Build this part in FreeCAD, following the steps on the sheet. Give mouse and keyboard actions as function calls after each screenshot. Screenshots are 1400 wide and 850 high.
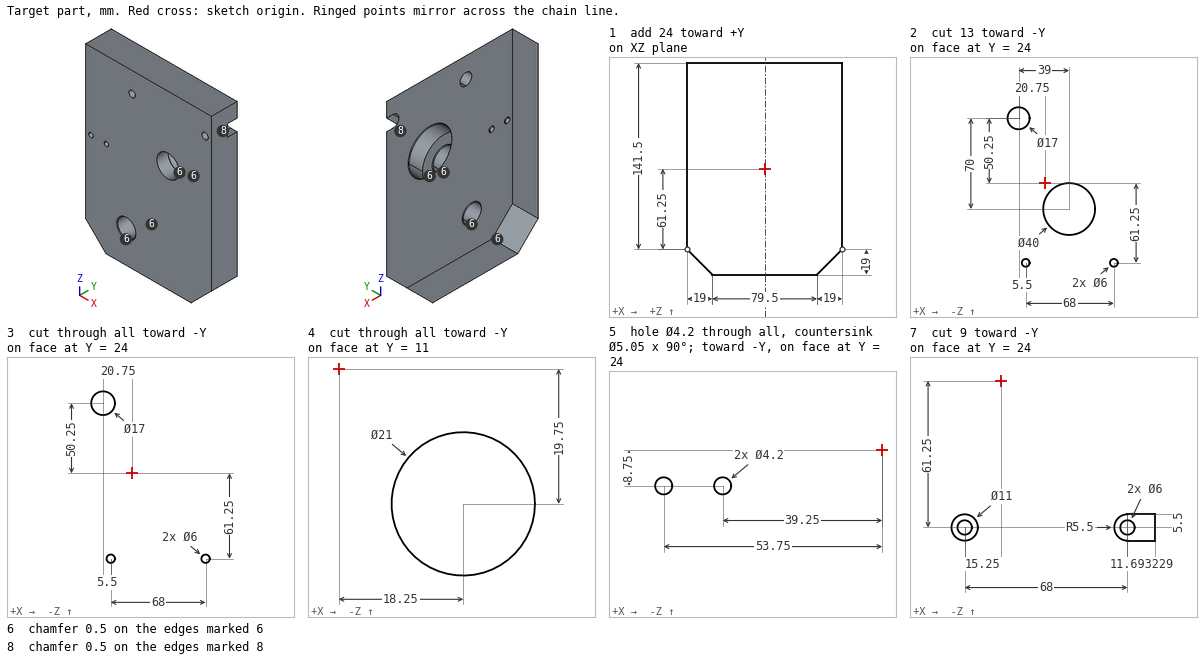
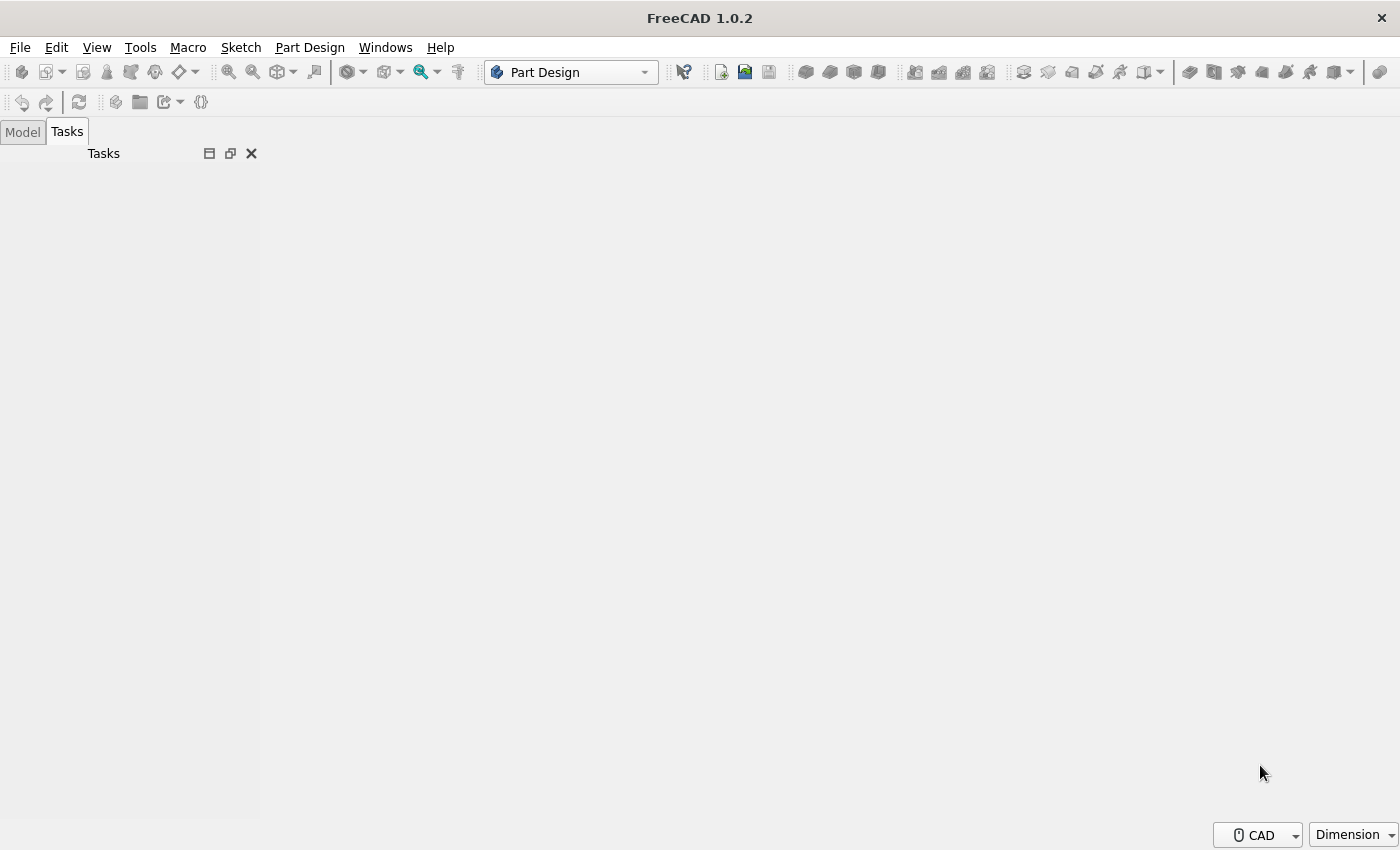
key(ctrl+n)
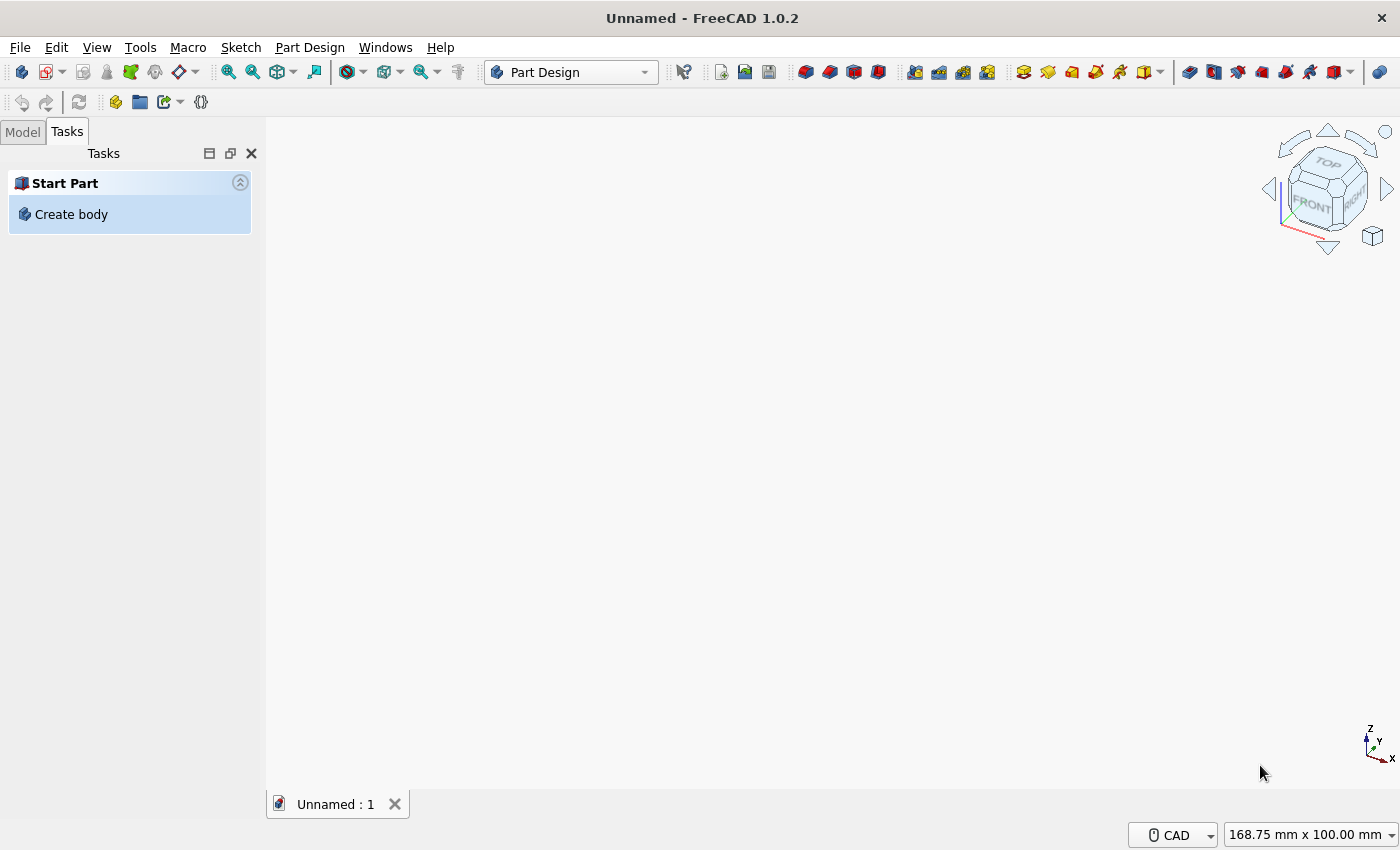
click(46, 72)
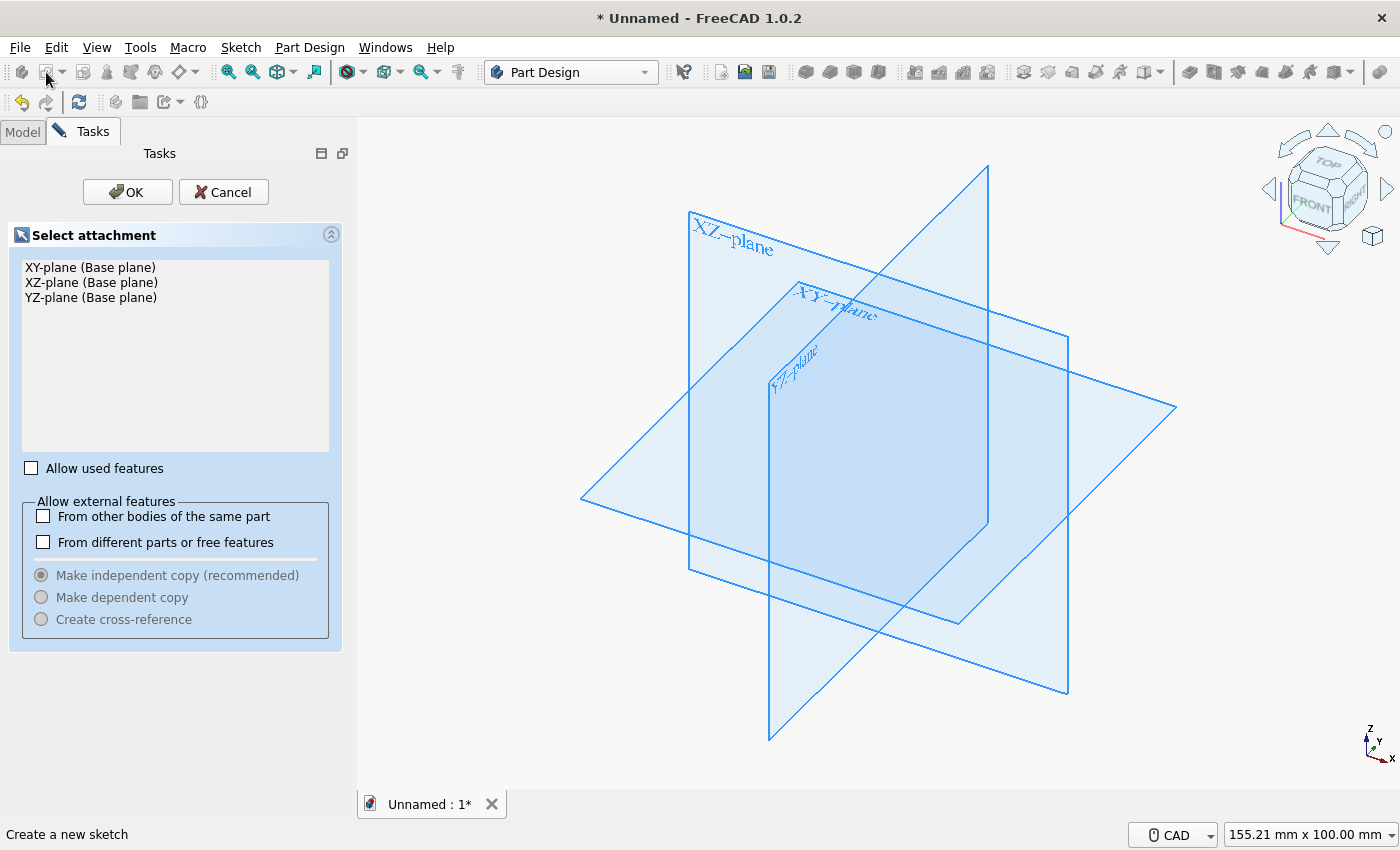
click(82, 282)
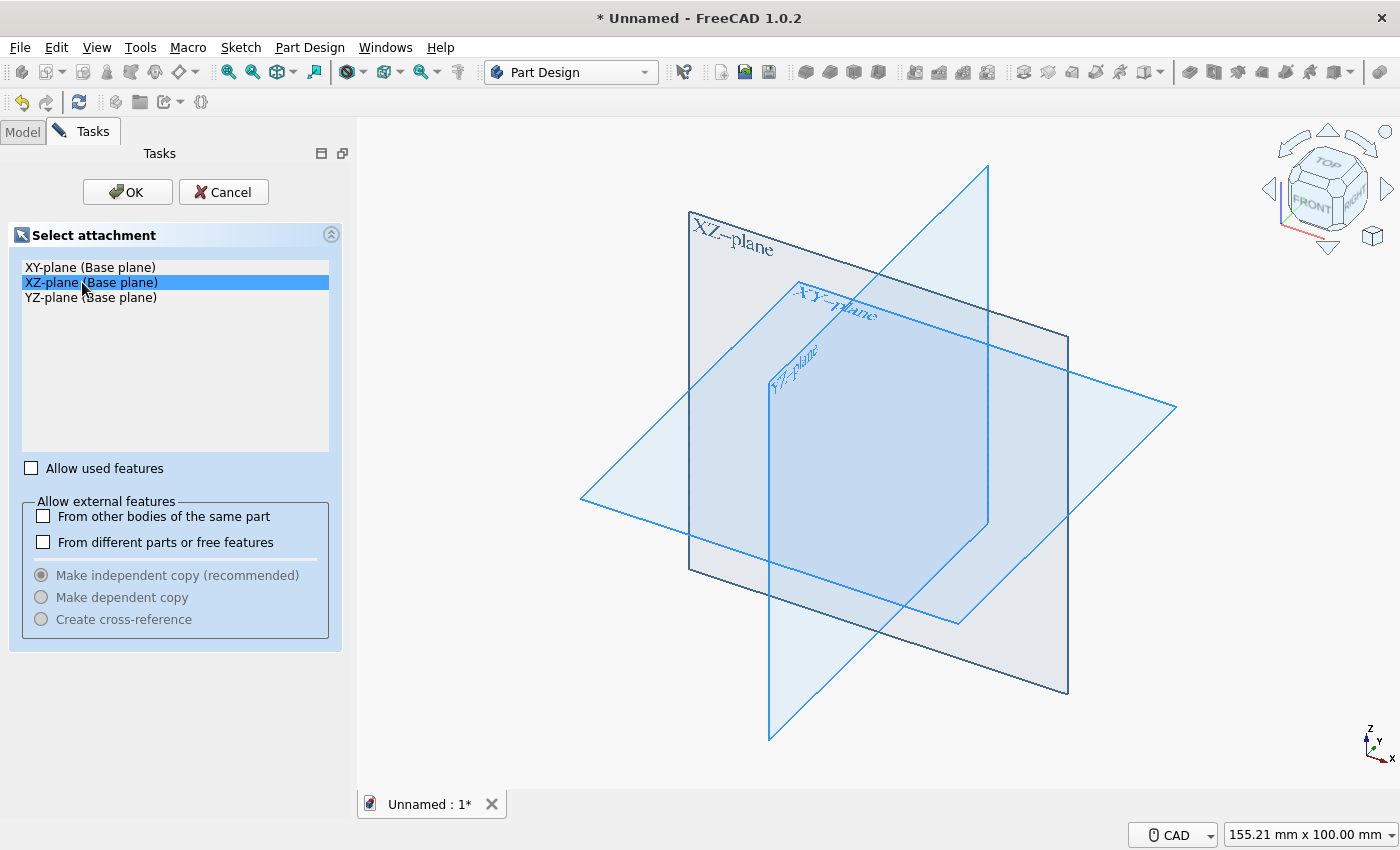
click(128, 192)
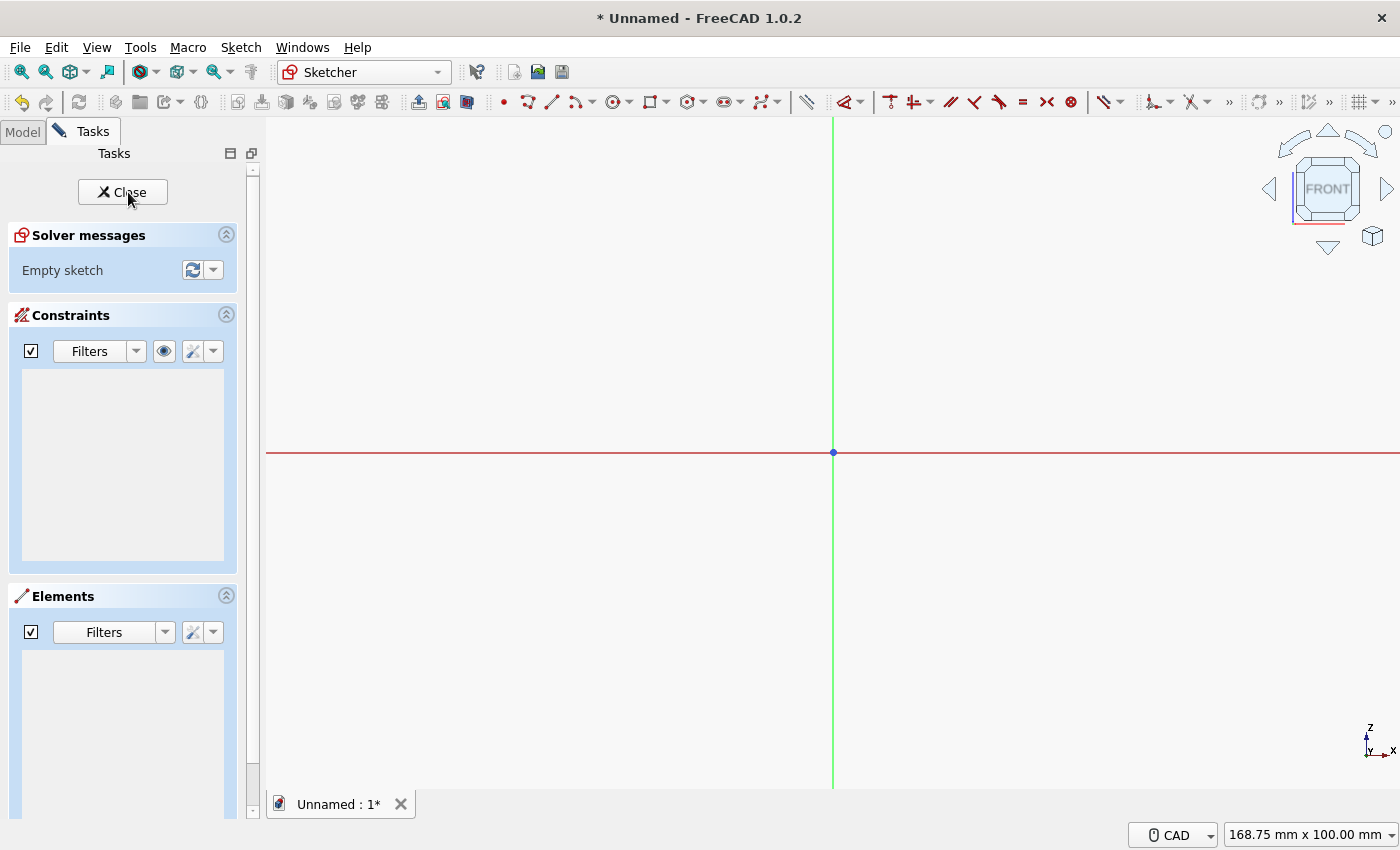
scroll(725, 453, down, 5)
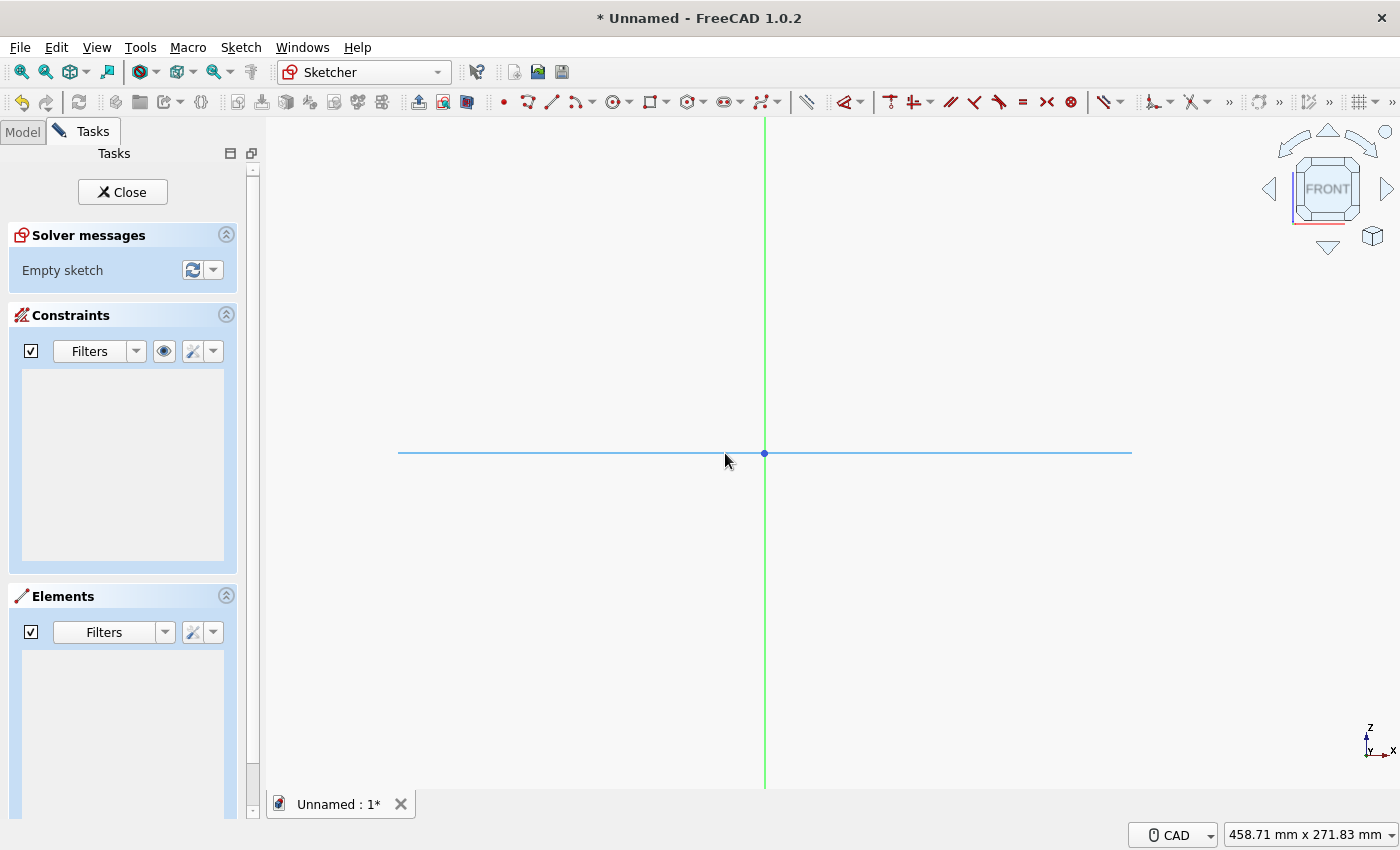
key(g)
key(m)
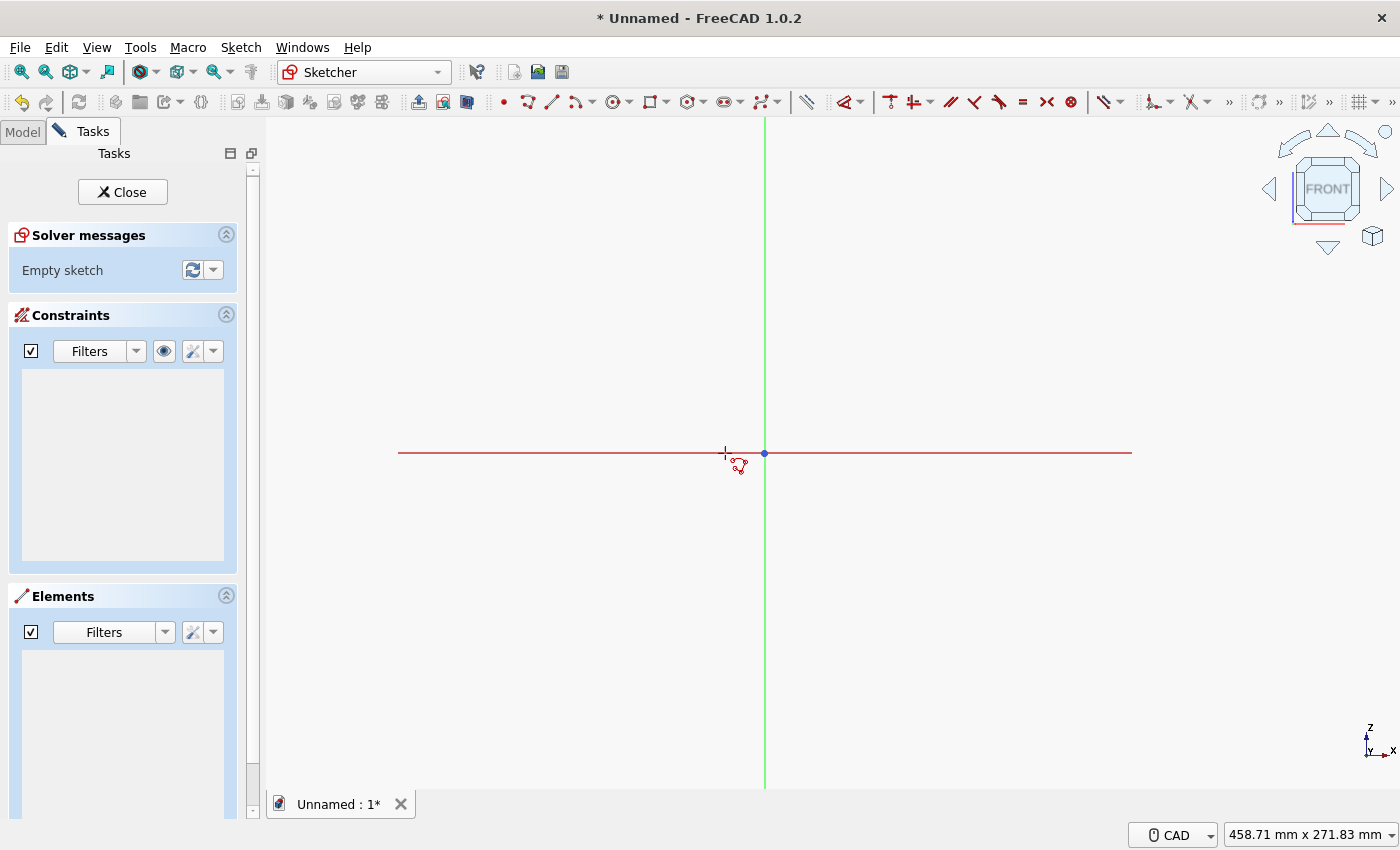
click(620, 605)
click(620, 255)
click(910, 255)
click(910, 605)
click(863, 652)
click(667, 652)
click(620, 606)
key(Escape)
key(Escape)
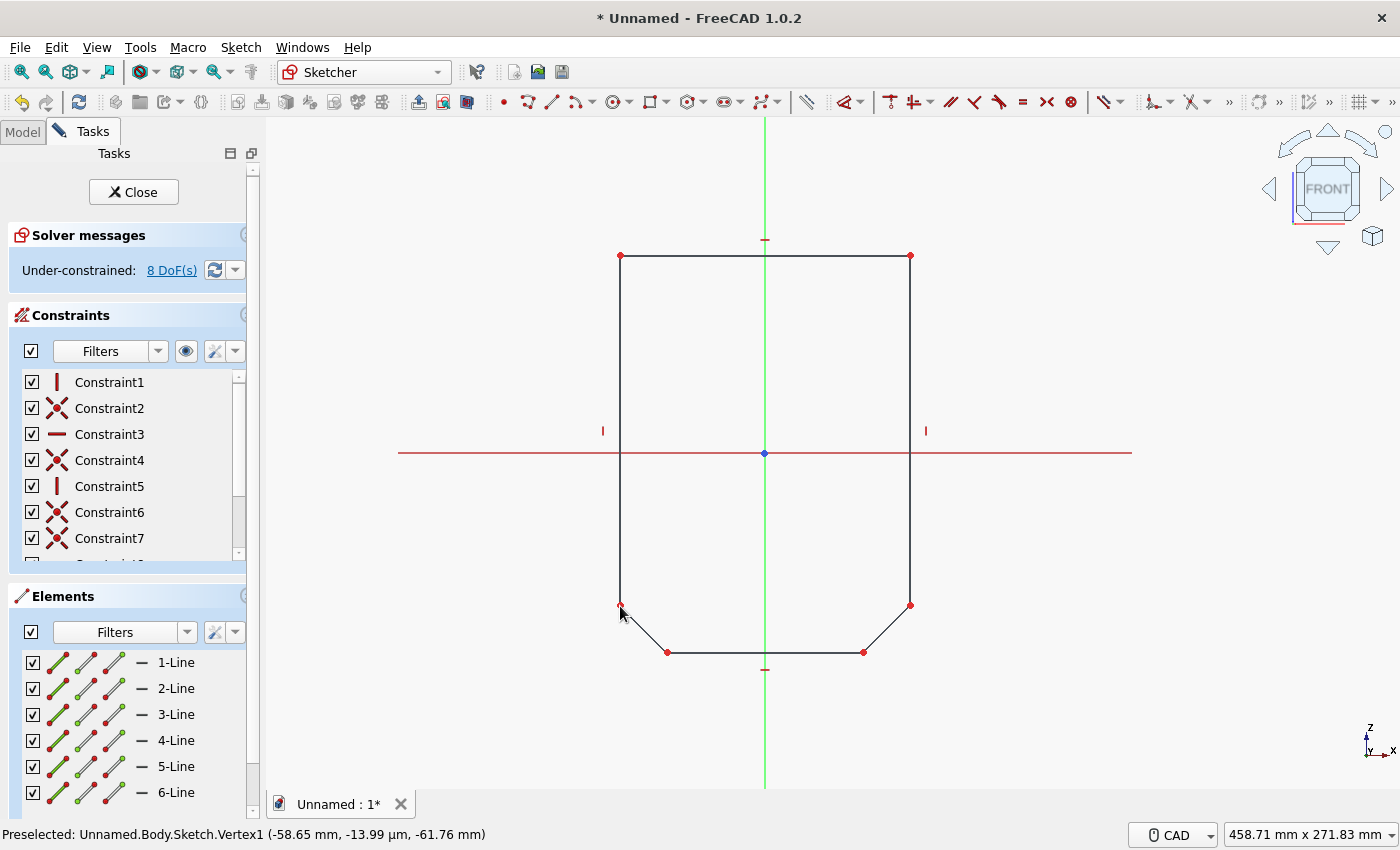
click(620, 606)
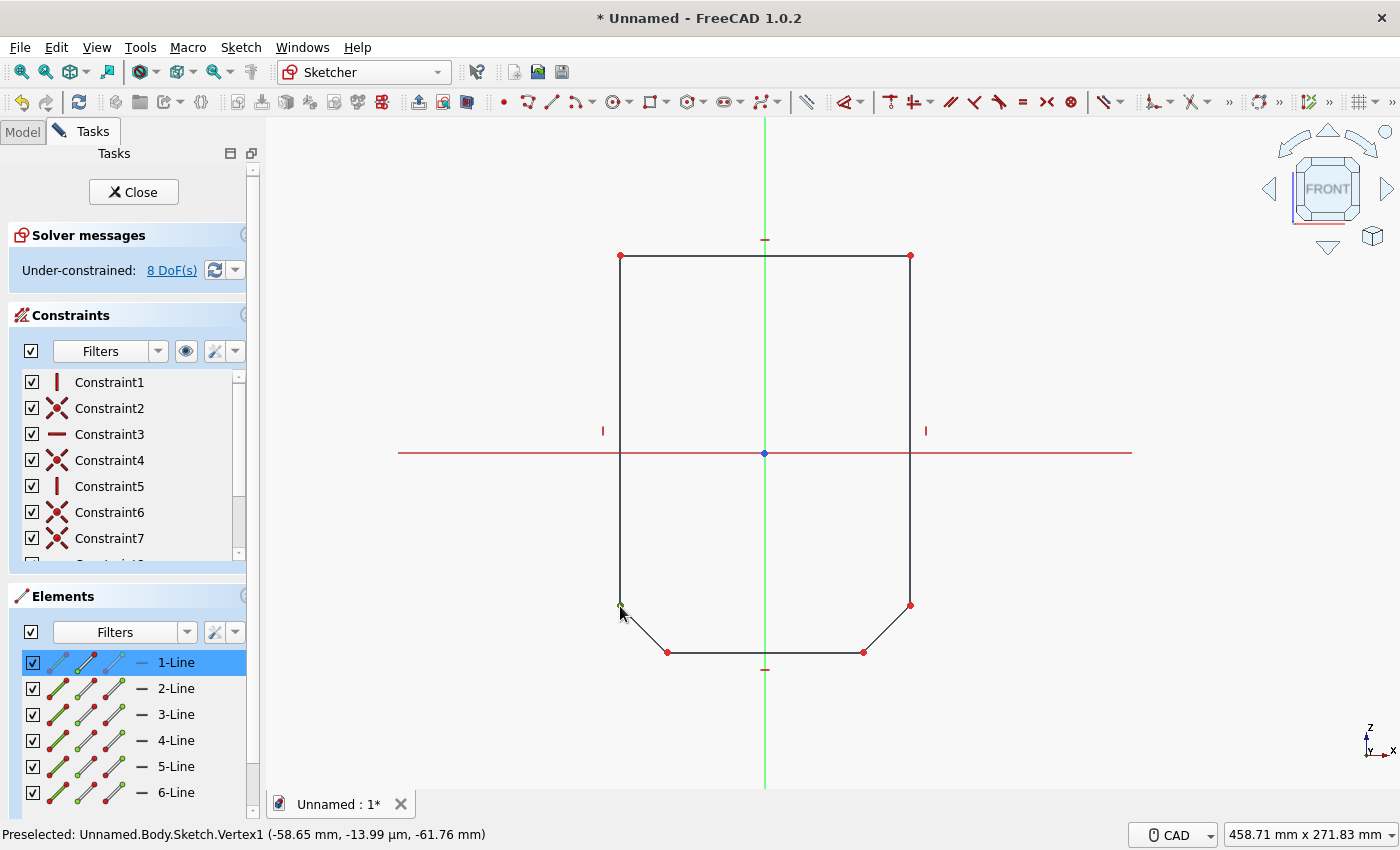
click(910, 606)